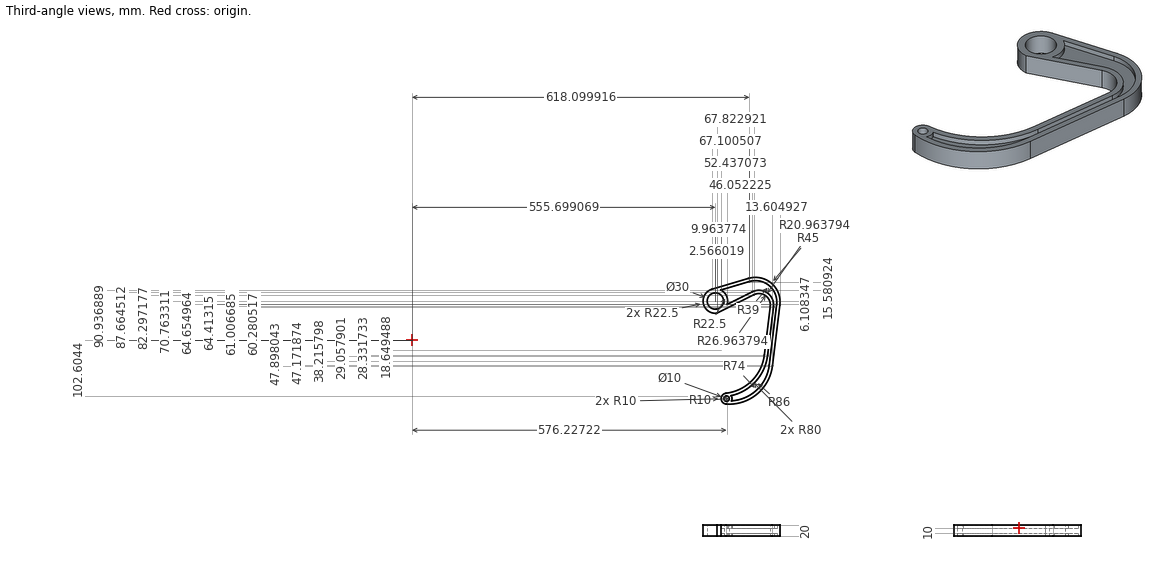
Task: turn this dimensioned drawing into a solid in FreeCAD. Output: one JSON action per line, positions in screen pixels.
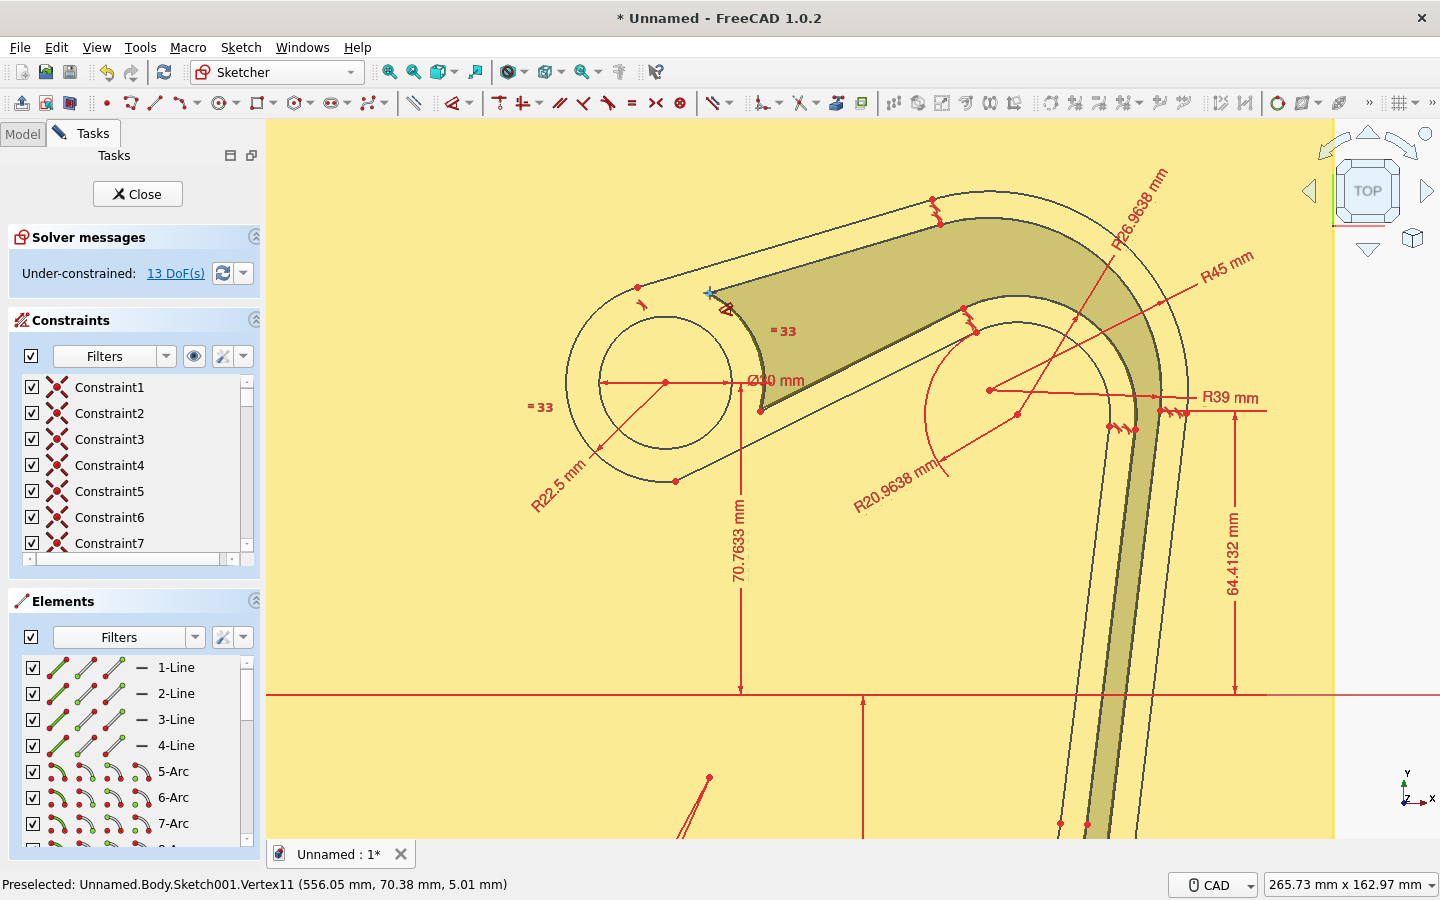
{"action": "left_click", "coordinate": [709, 293]}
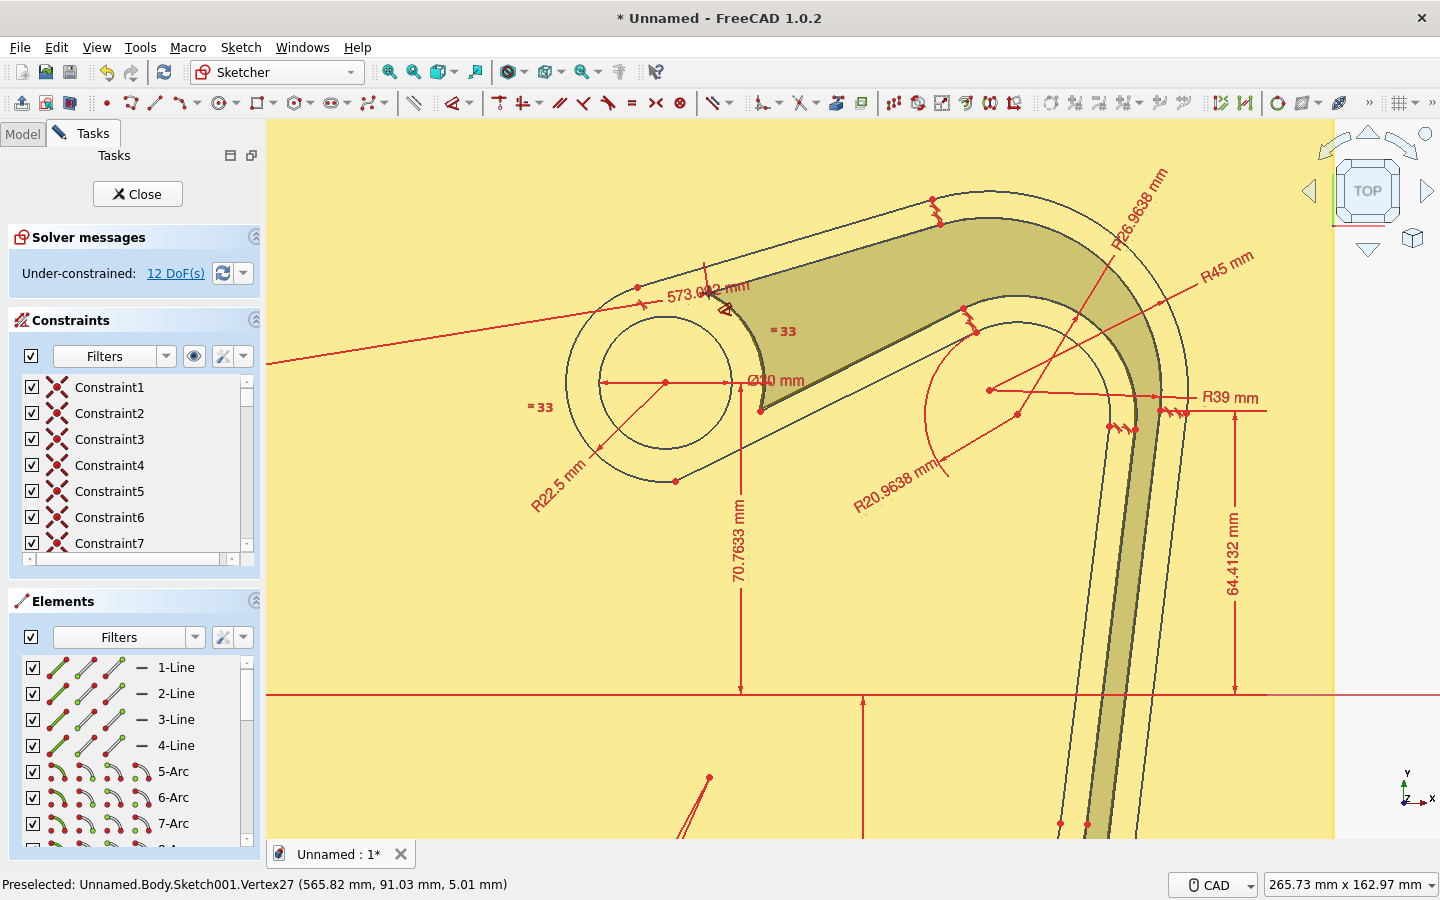
{"action": "left_click", "coordinate": [666, 383]}
{"action": "left_click", "coordinate": [677, 259]}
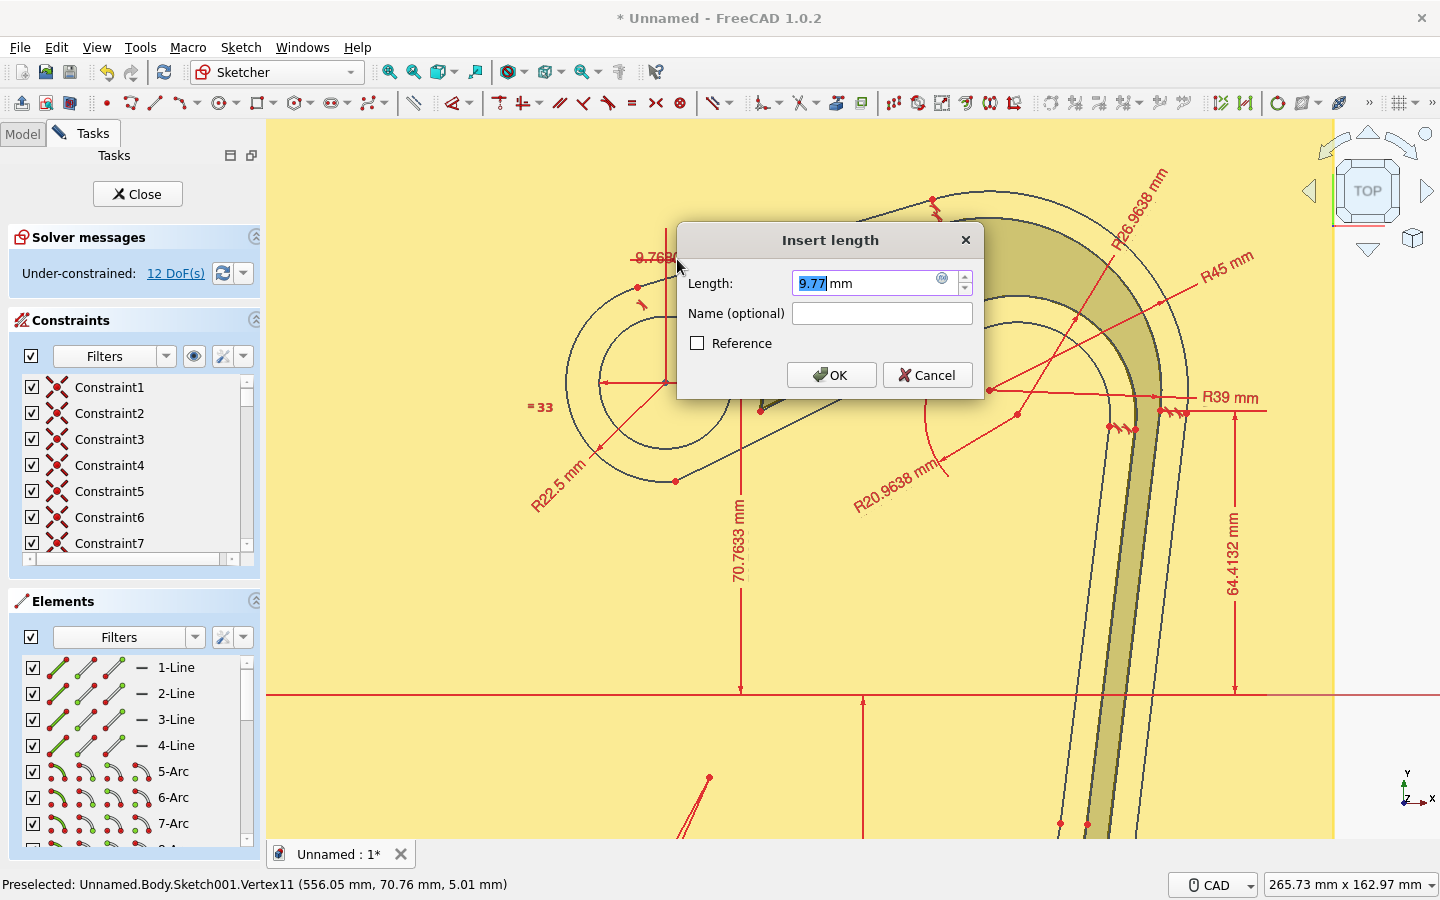
{"action": "type", "text": "9.963774"}
{"action": "key", "text": "Return"}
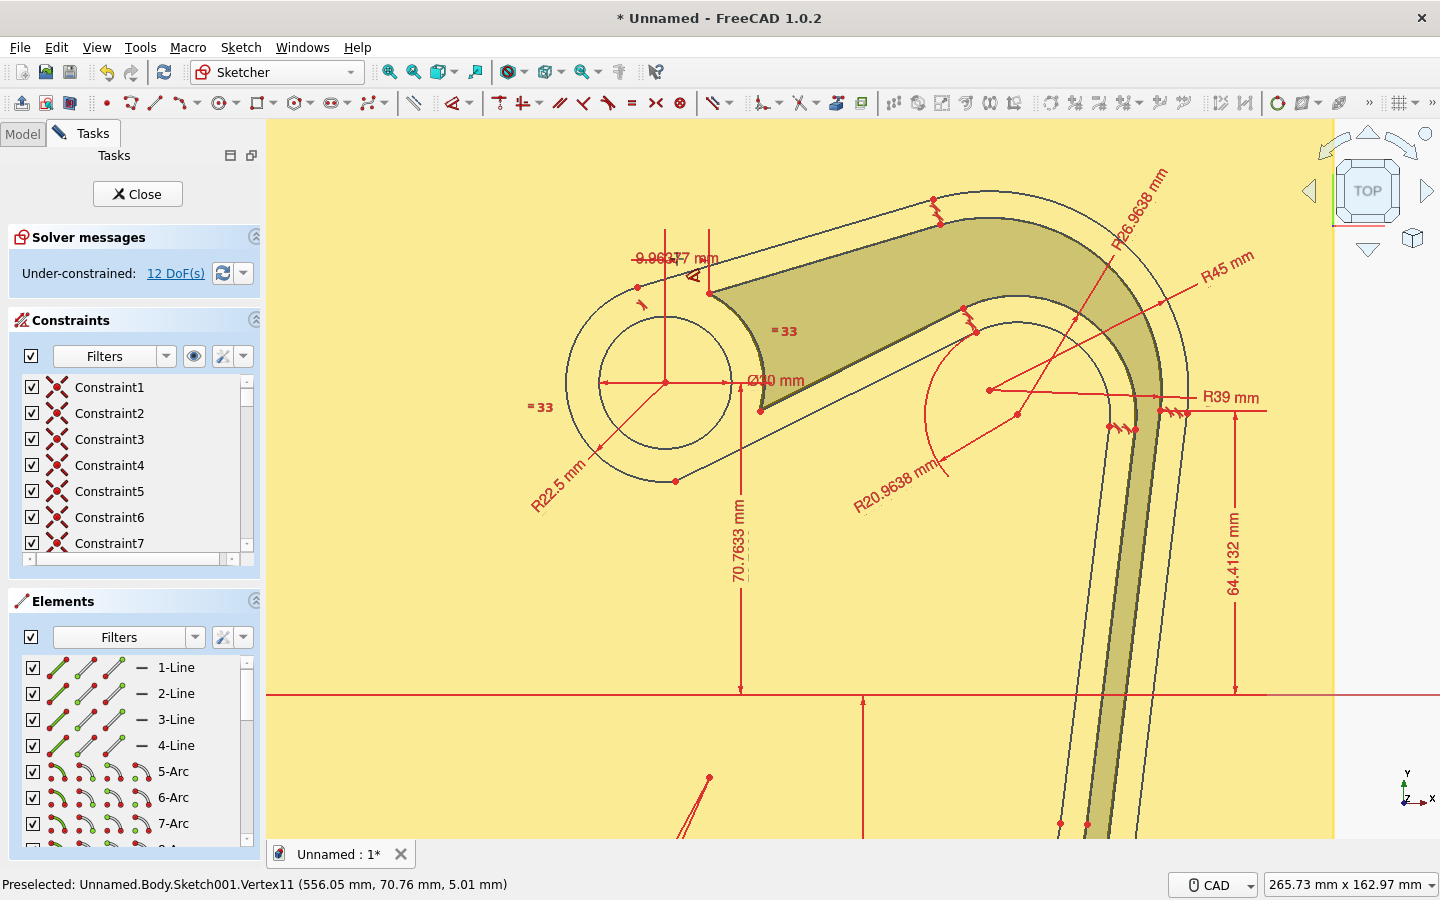
{"action": "scroll", "coordinate": [675, 482], "scroll_direction": "up", "scroll_amount": 7}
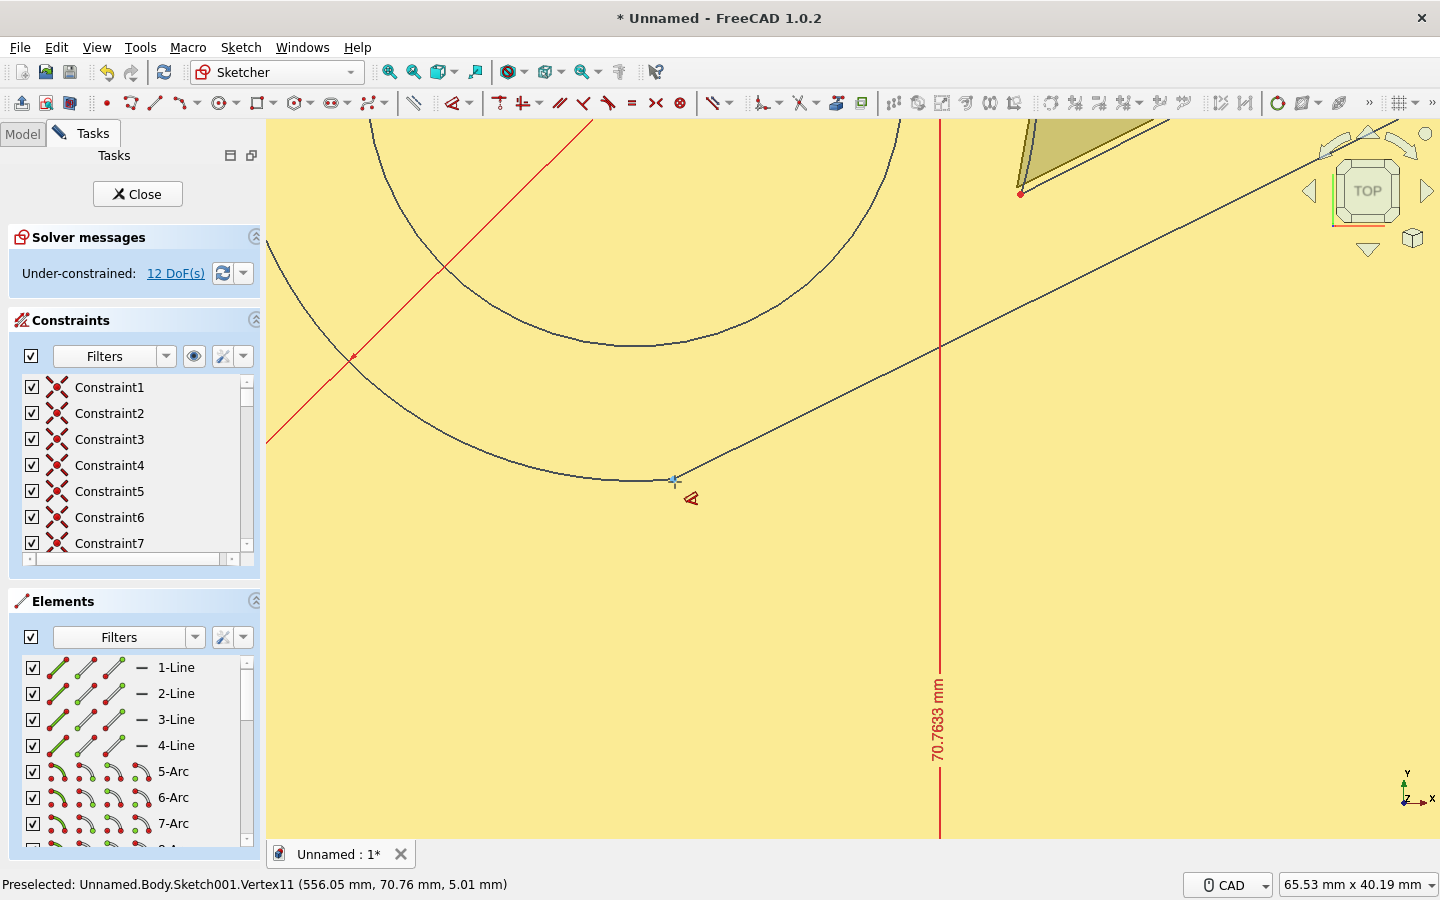
{"action": "left_click", "coordinate": [674, 479]}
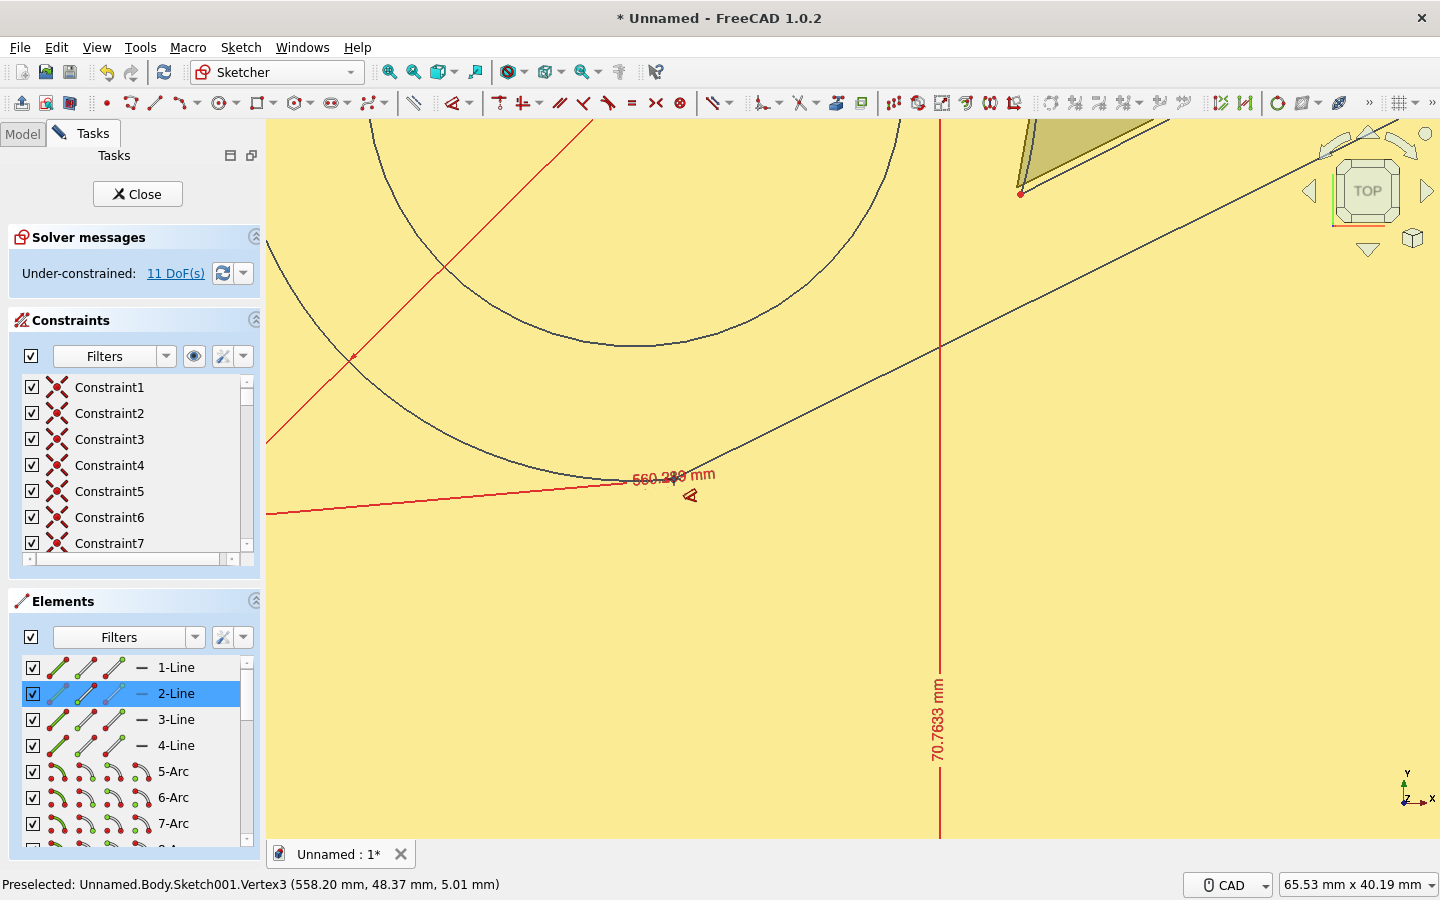
{"action": "scroll", "coordinate": [697, 365], "scroll_direction": "down", "scroll_amount": 11}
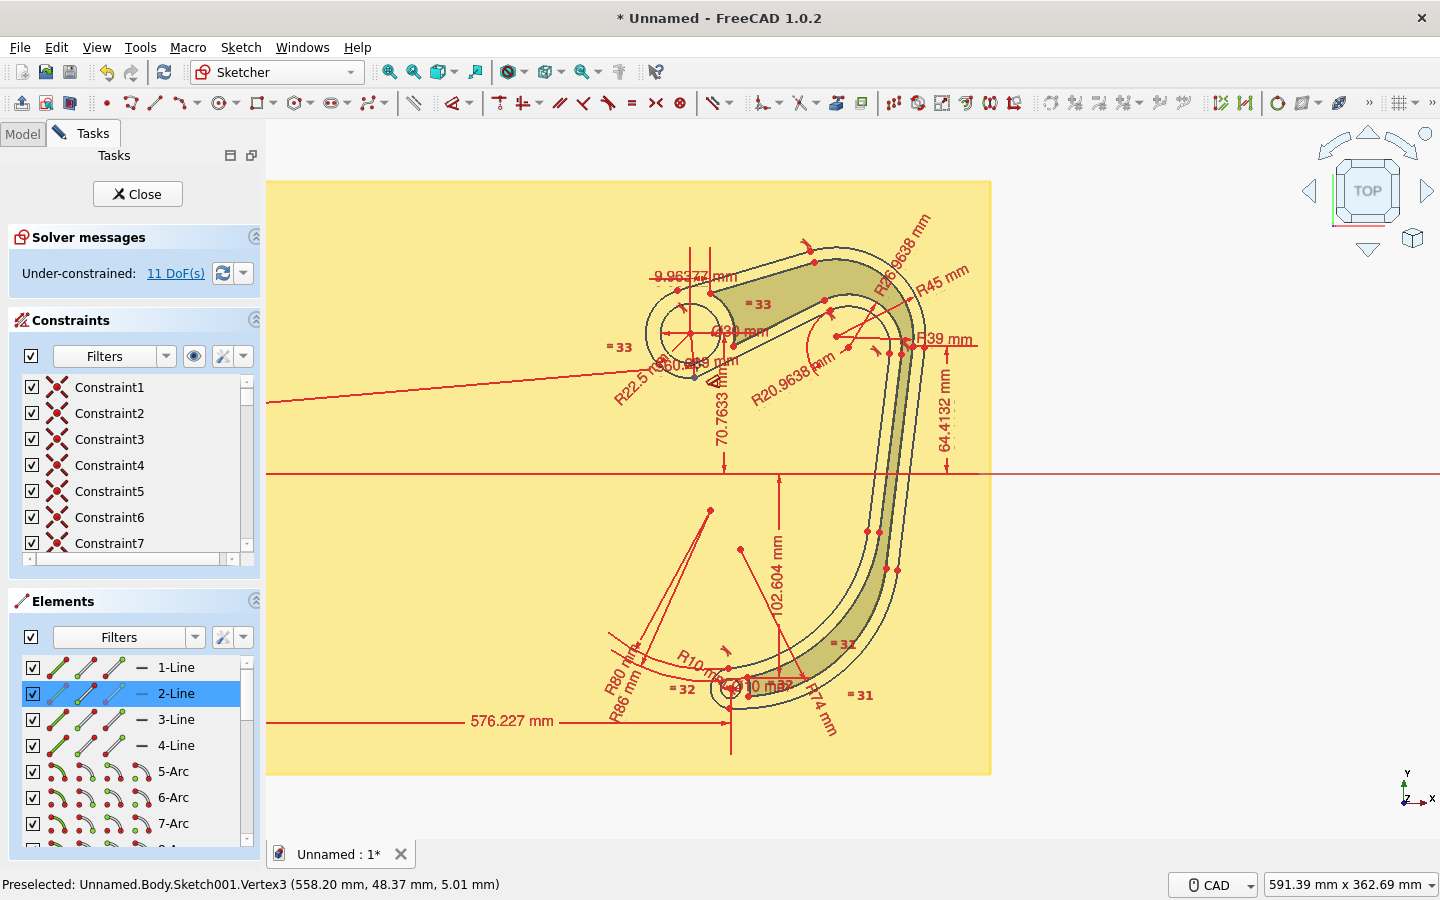
{"action": "scroll", "coordinate": [690, 333], "scroll_direction": "up", "scroll_amount": 11}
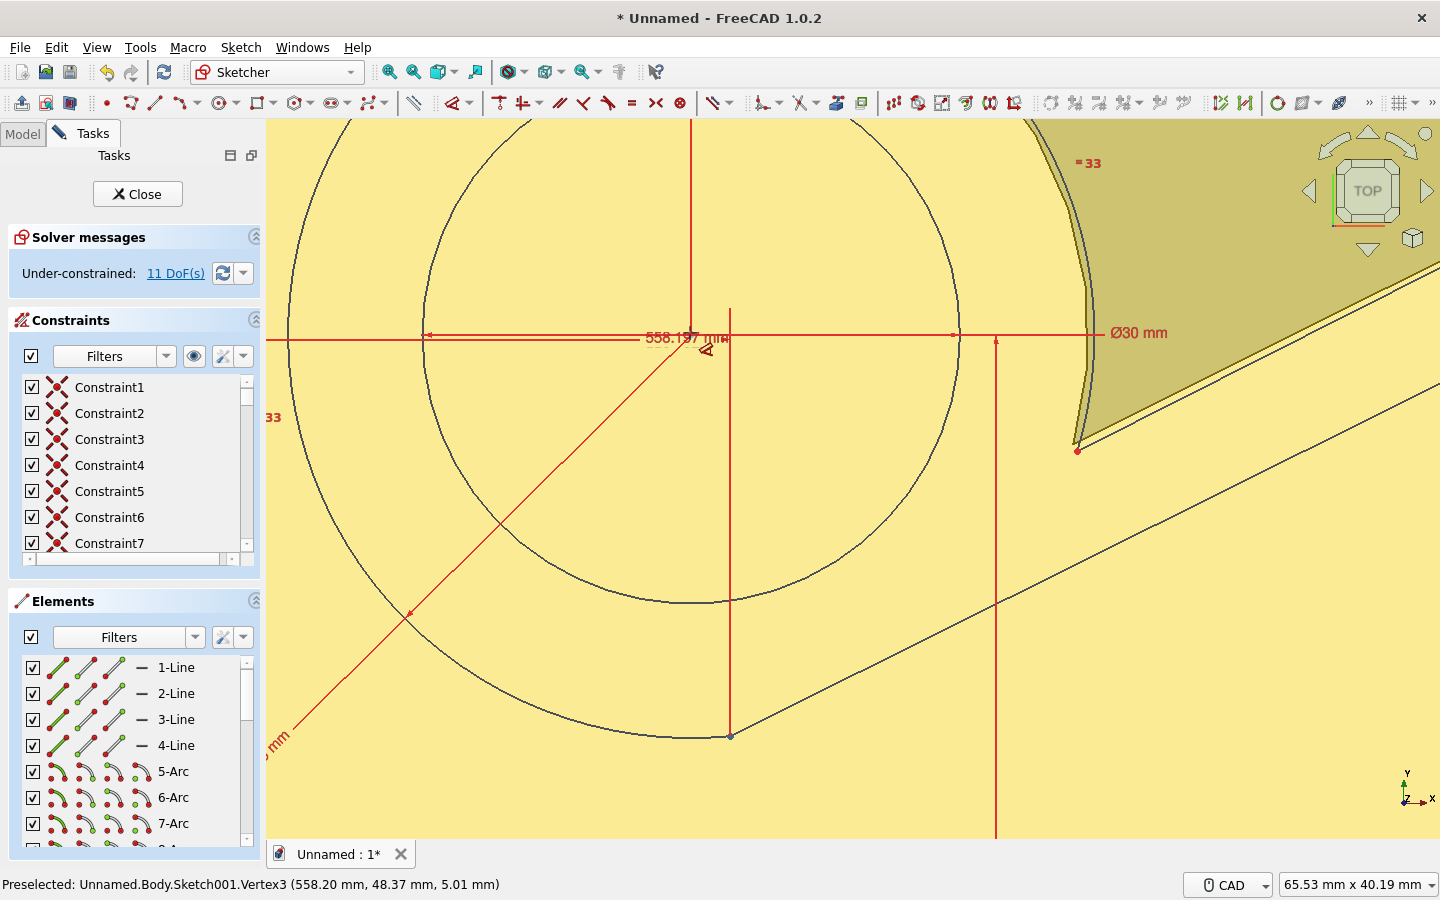
{"action": "left_click", "coordinate": [691, 335]}
{"action": "left_click", "coordinate": [711, 301]}